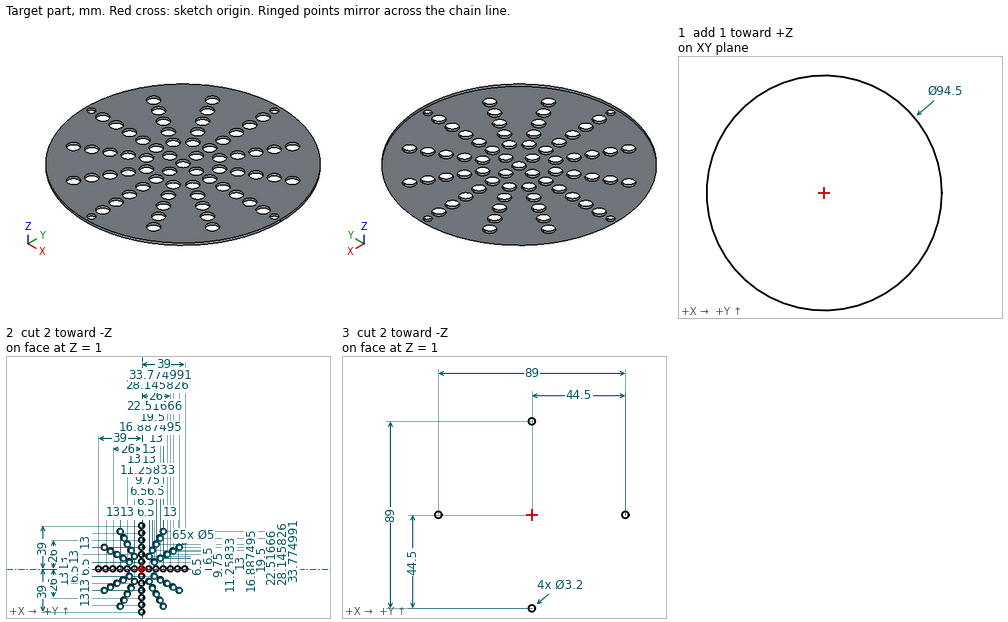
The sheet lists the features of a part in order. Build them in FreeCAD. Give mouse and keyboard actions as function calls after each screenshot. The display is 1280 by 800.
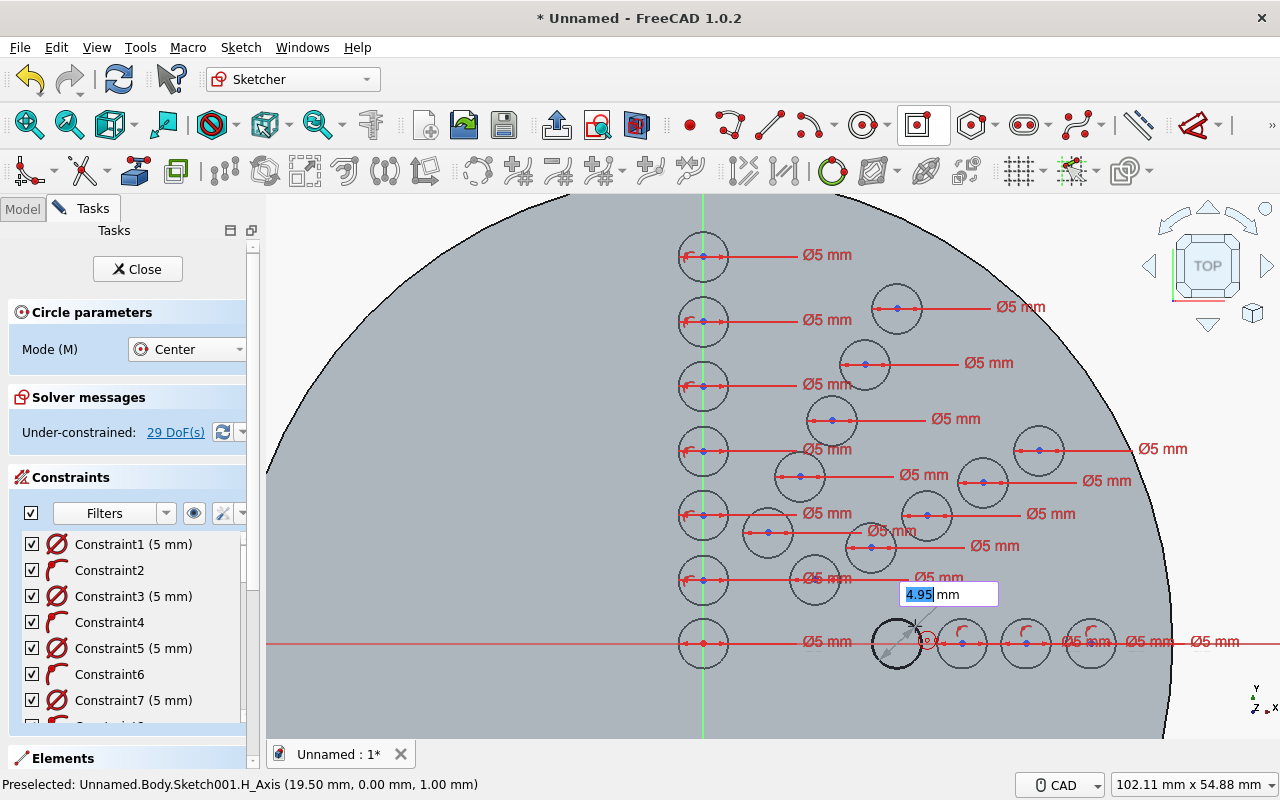
text(5)
key(Return)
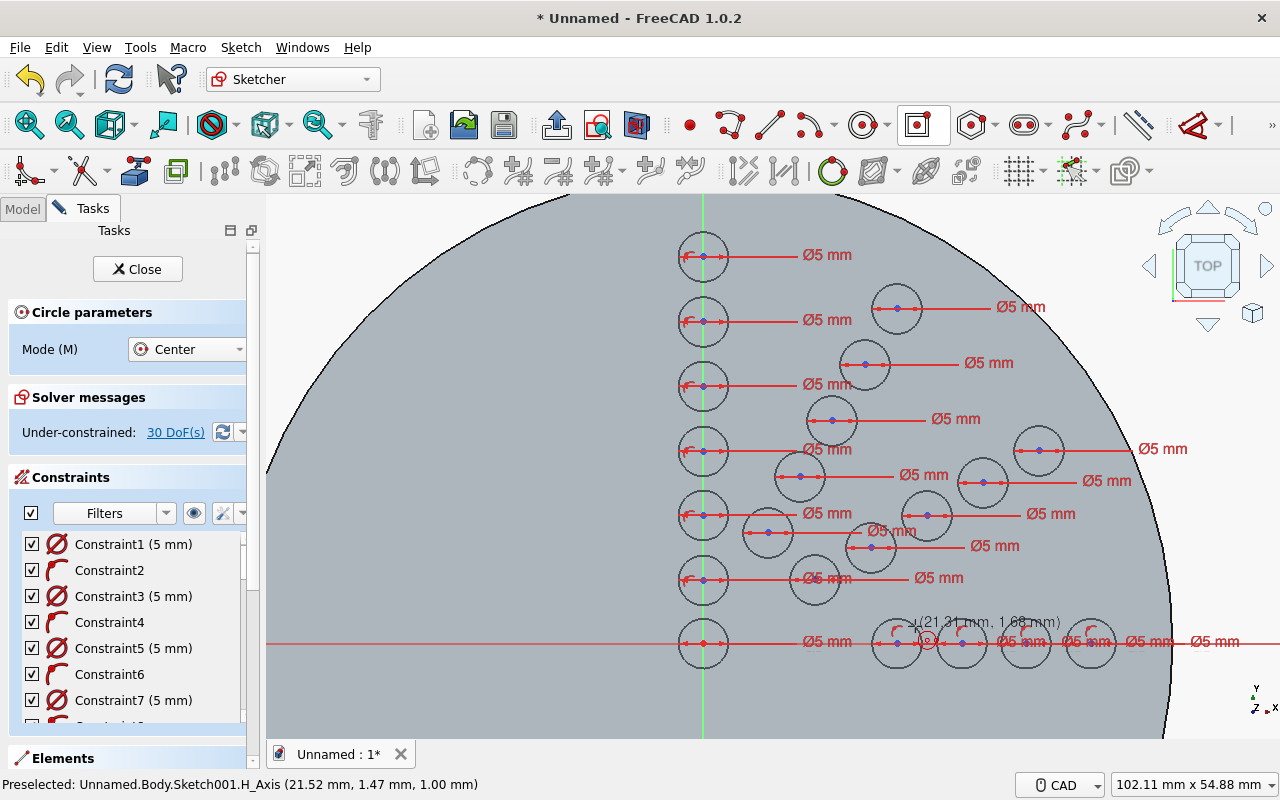
click(832, 644)
move(850, 626)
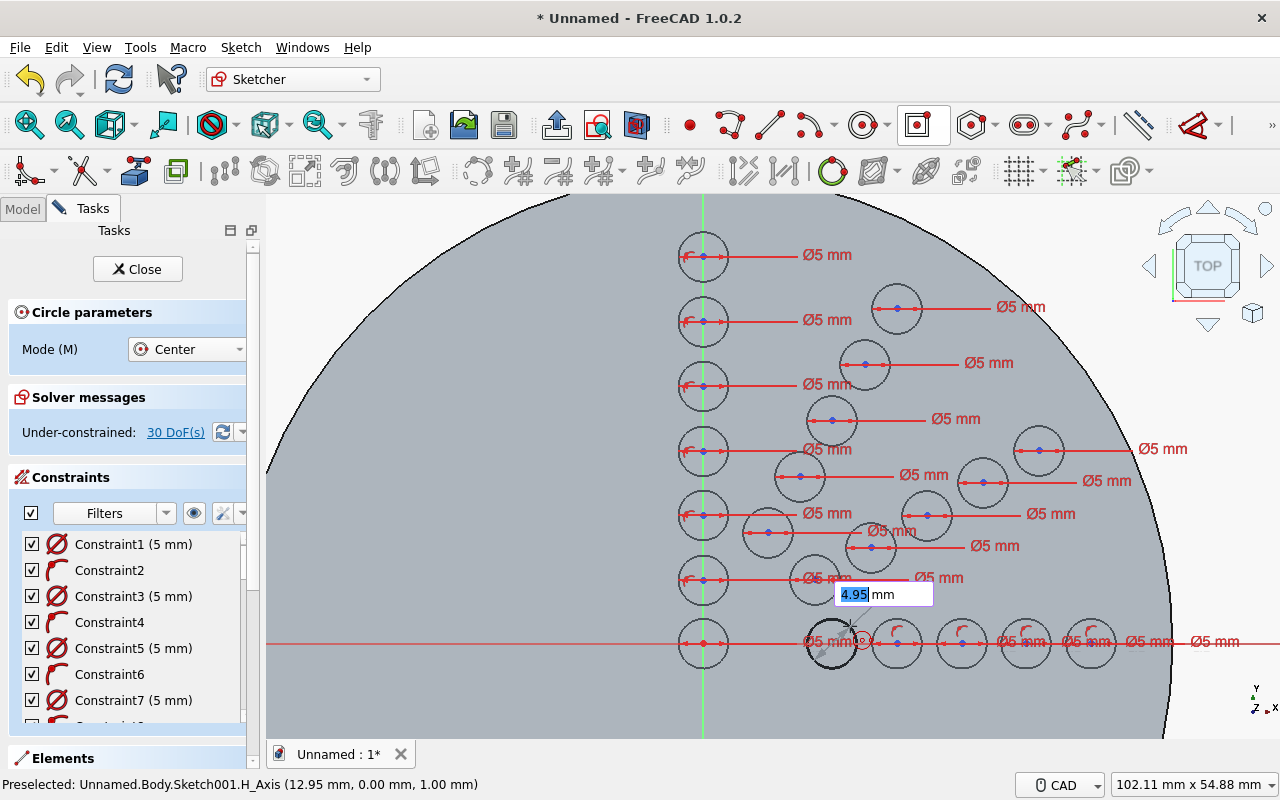
text(5)
key(Return)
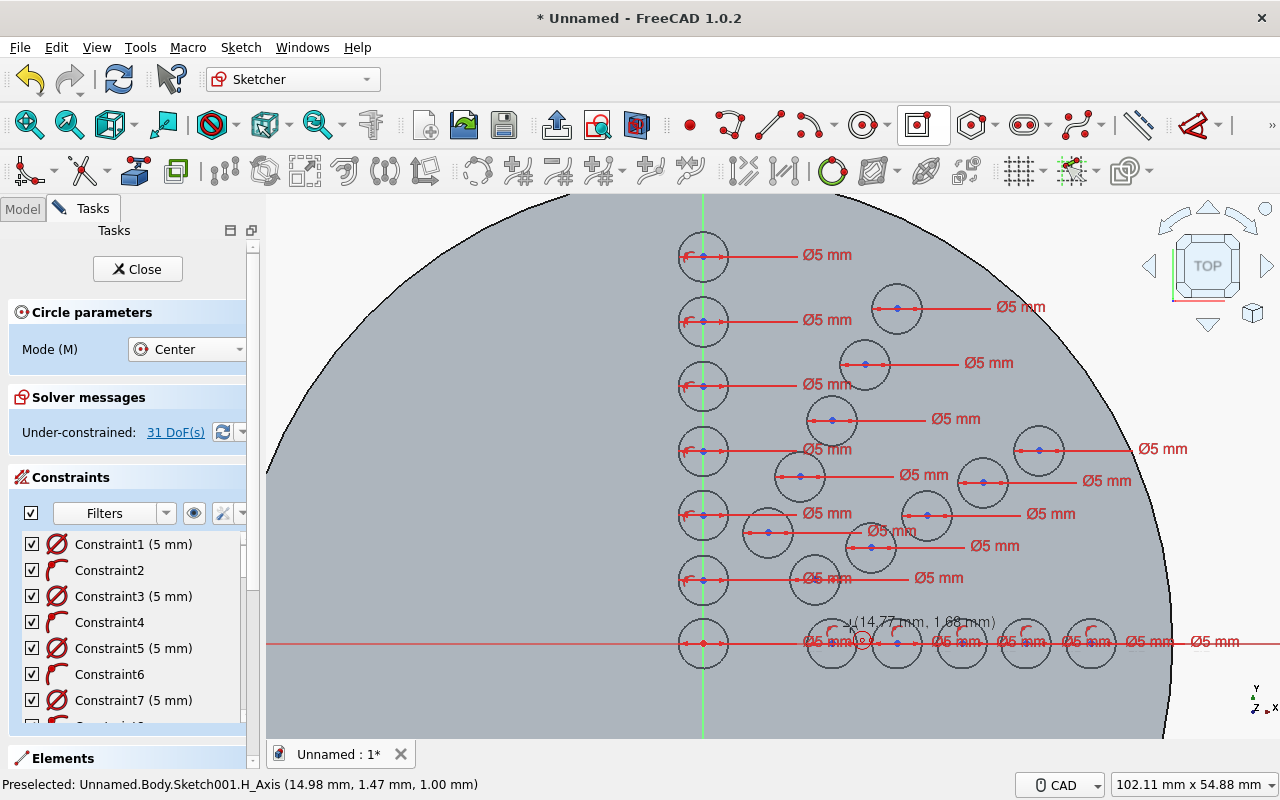
scroll(705, 322, down, 4)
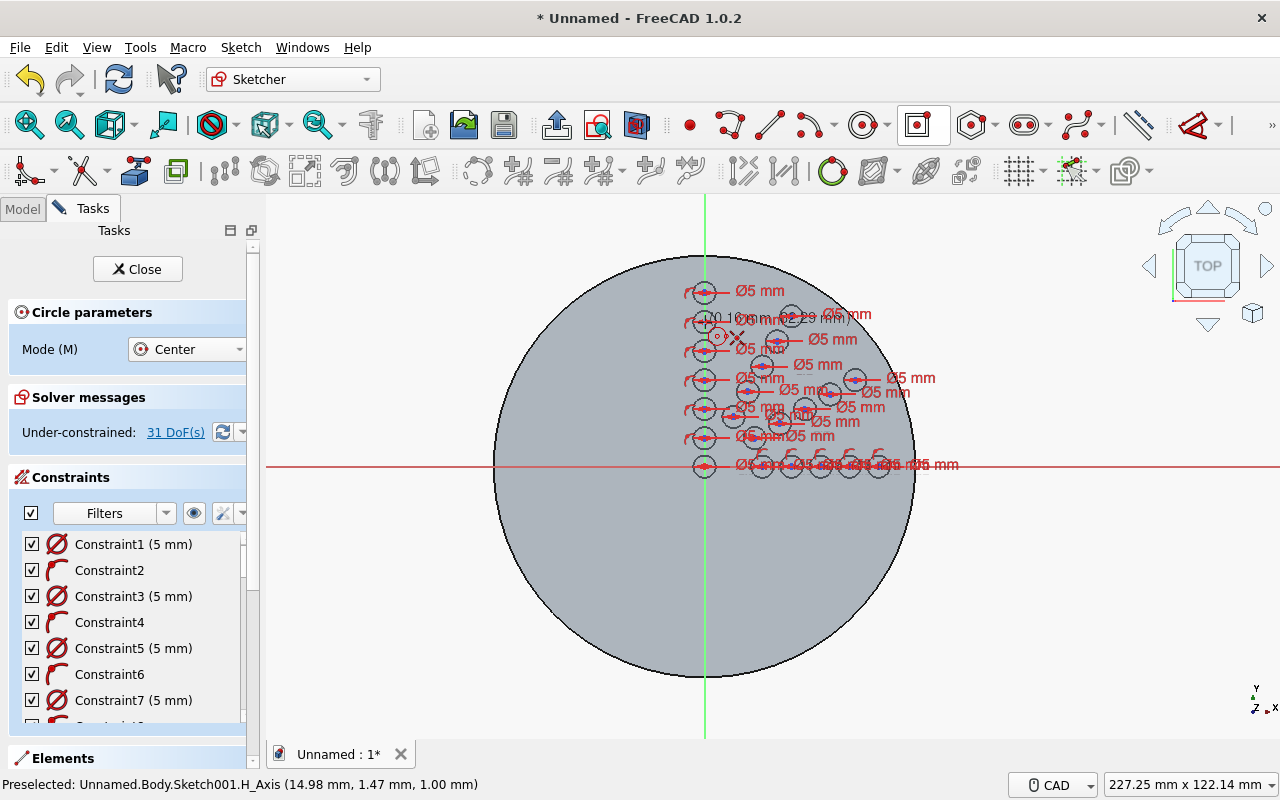
scroll(855, 554, up, 4)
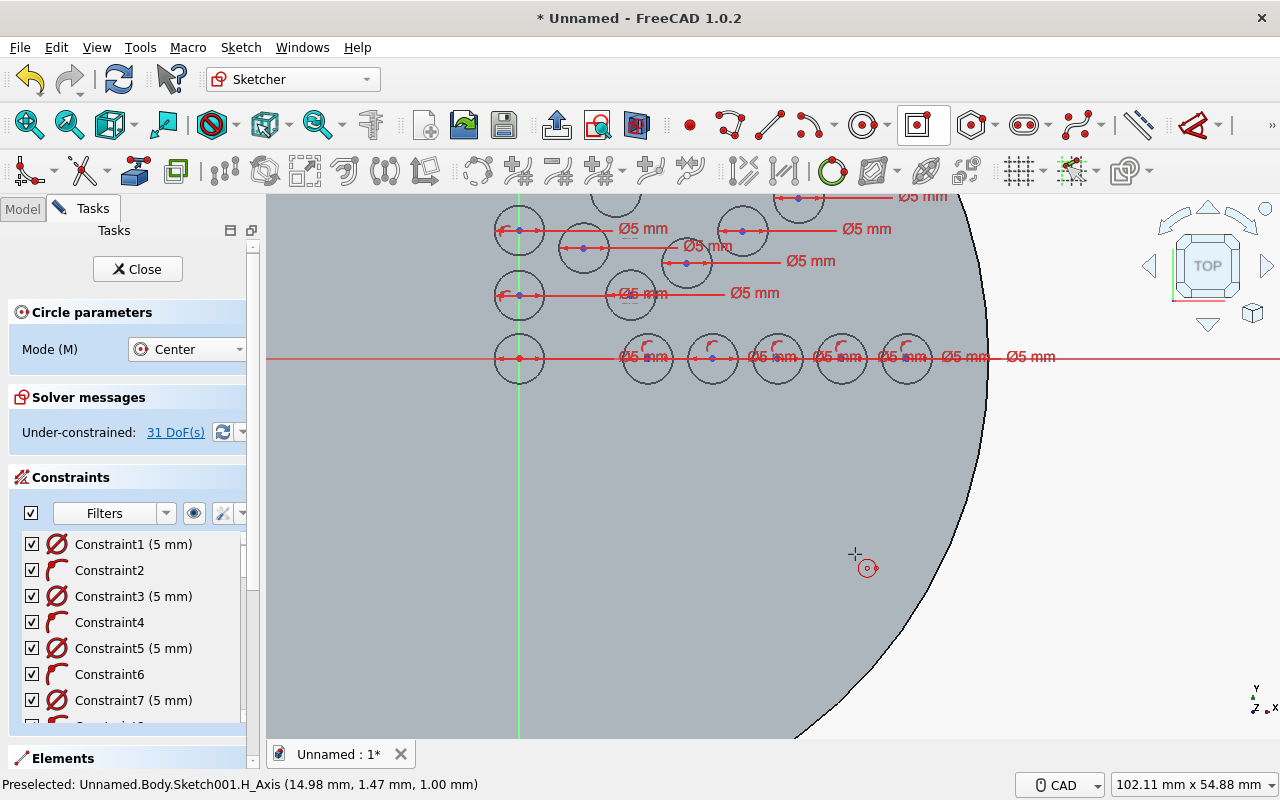
click(855, 553)
move(872, 535)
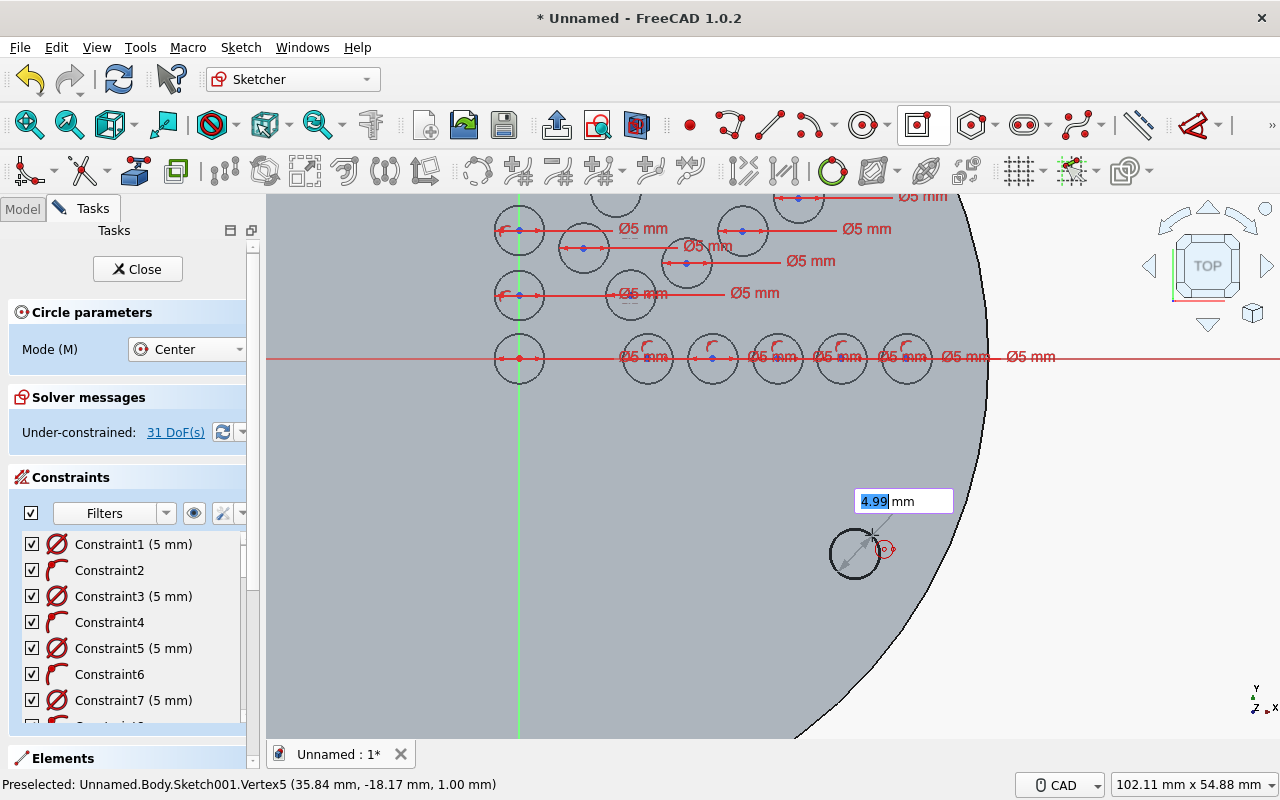
text(5)
key(Return)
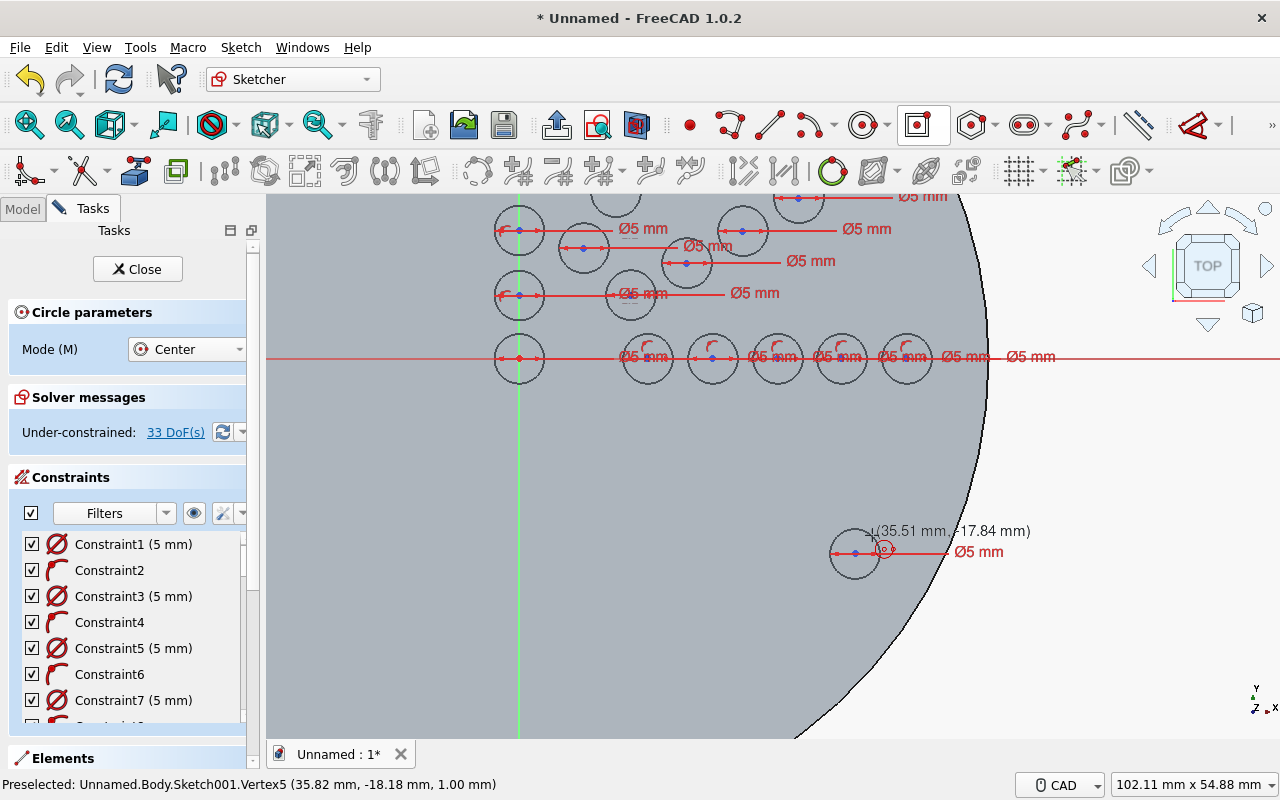
click(799, 520)
move(816, 503)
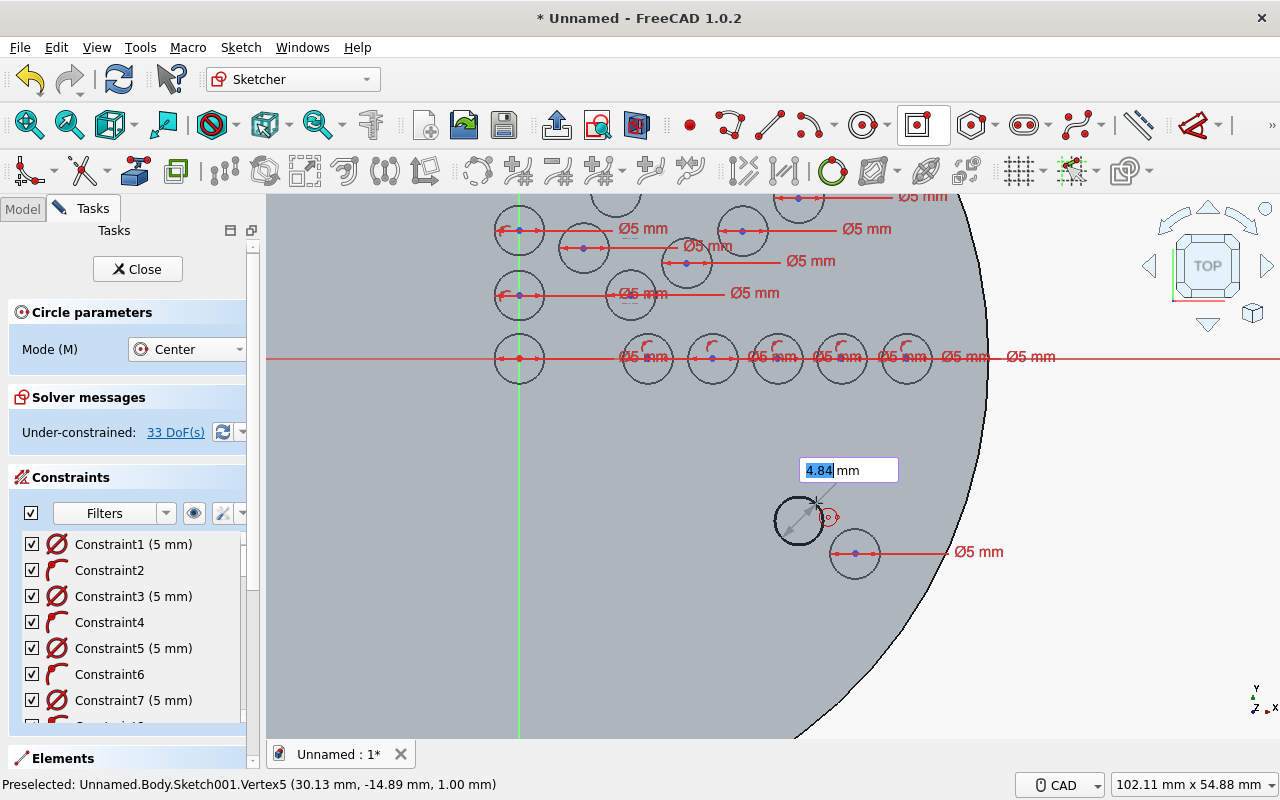
text(5)
key(Return)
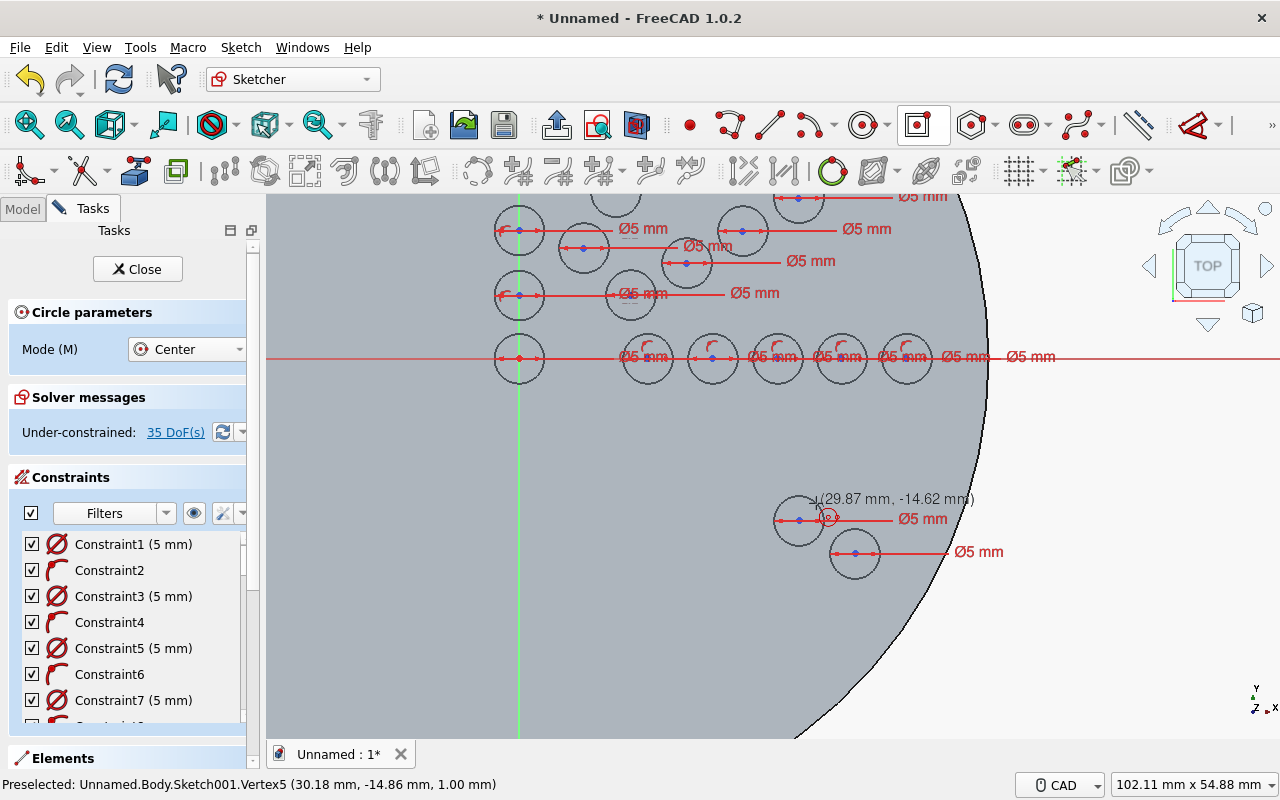
click(743, 488)
move(761, 470)